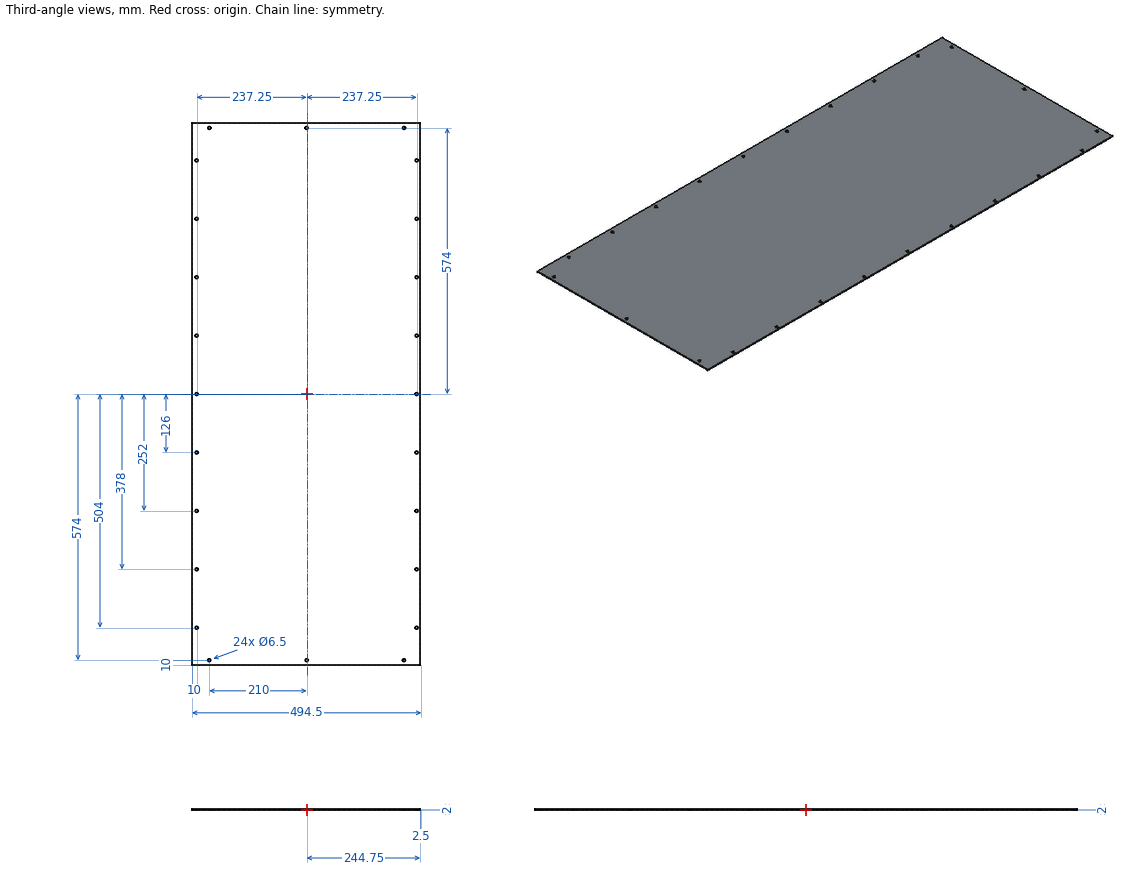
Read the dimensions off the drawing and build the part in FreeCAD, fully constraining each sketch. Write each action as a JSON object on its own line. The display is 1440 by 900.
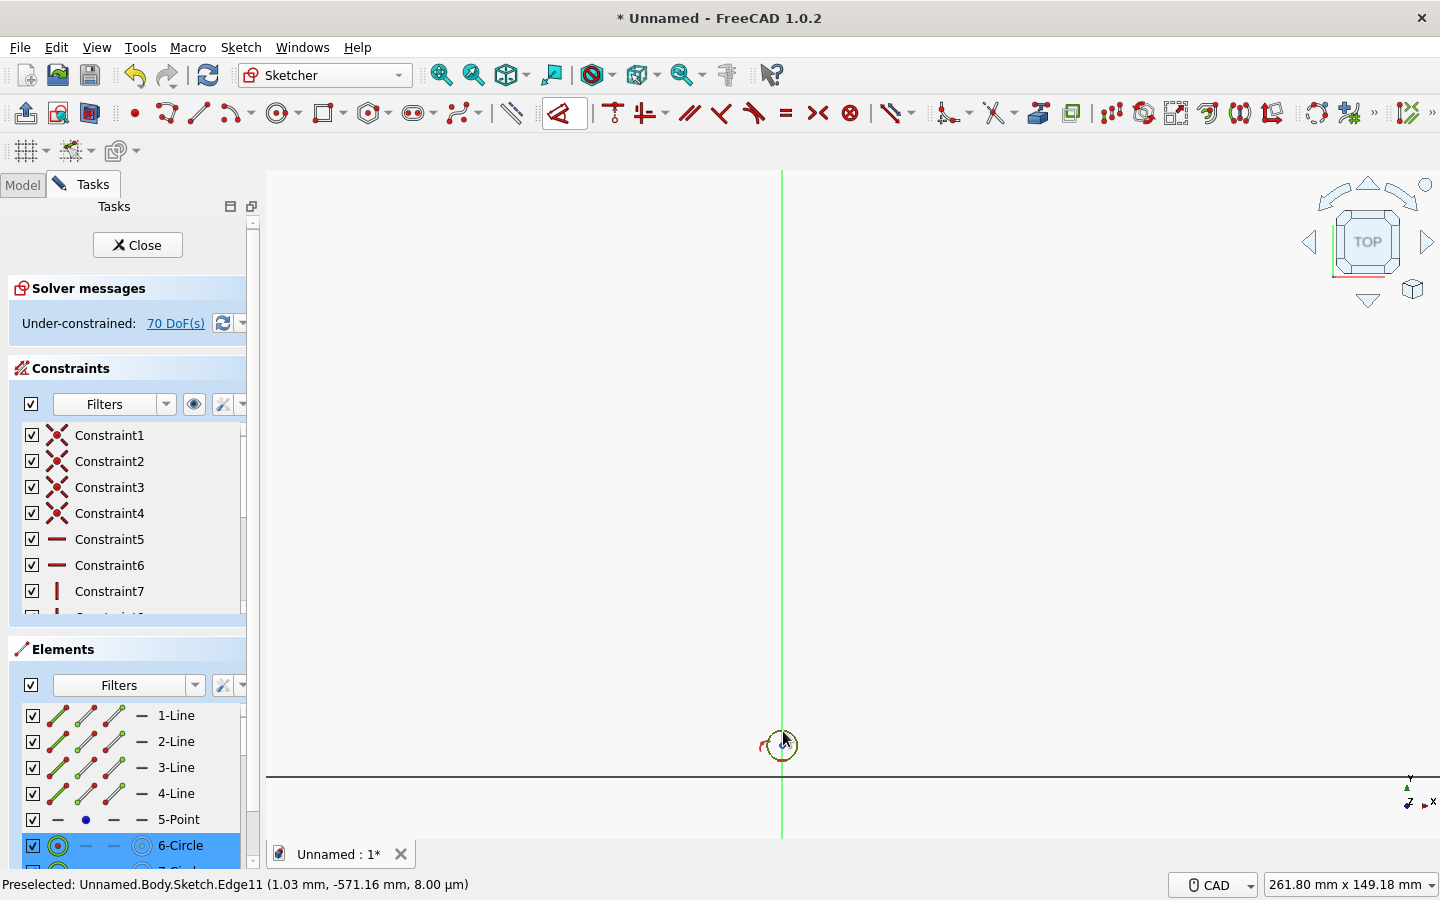
{"action": "scroll", "coordinate": [785, 737], "scroll_direction": "down", "scroll_amount": 12}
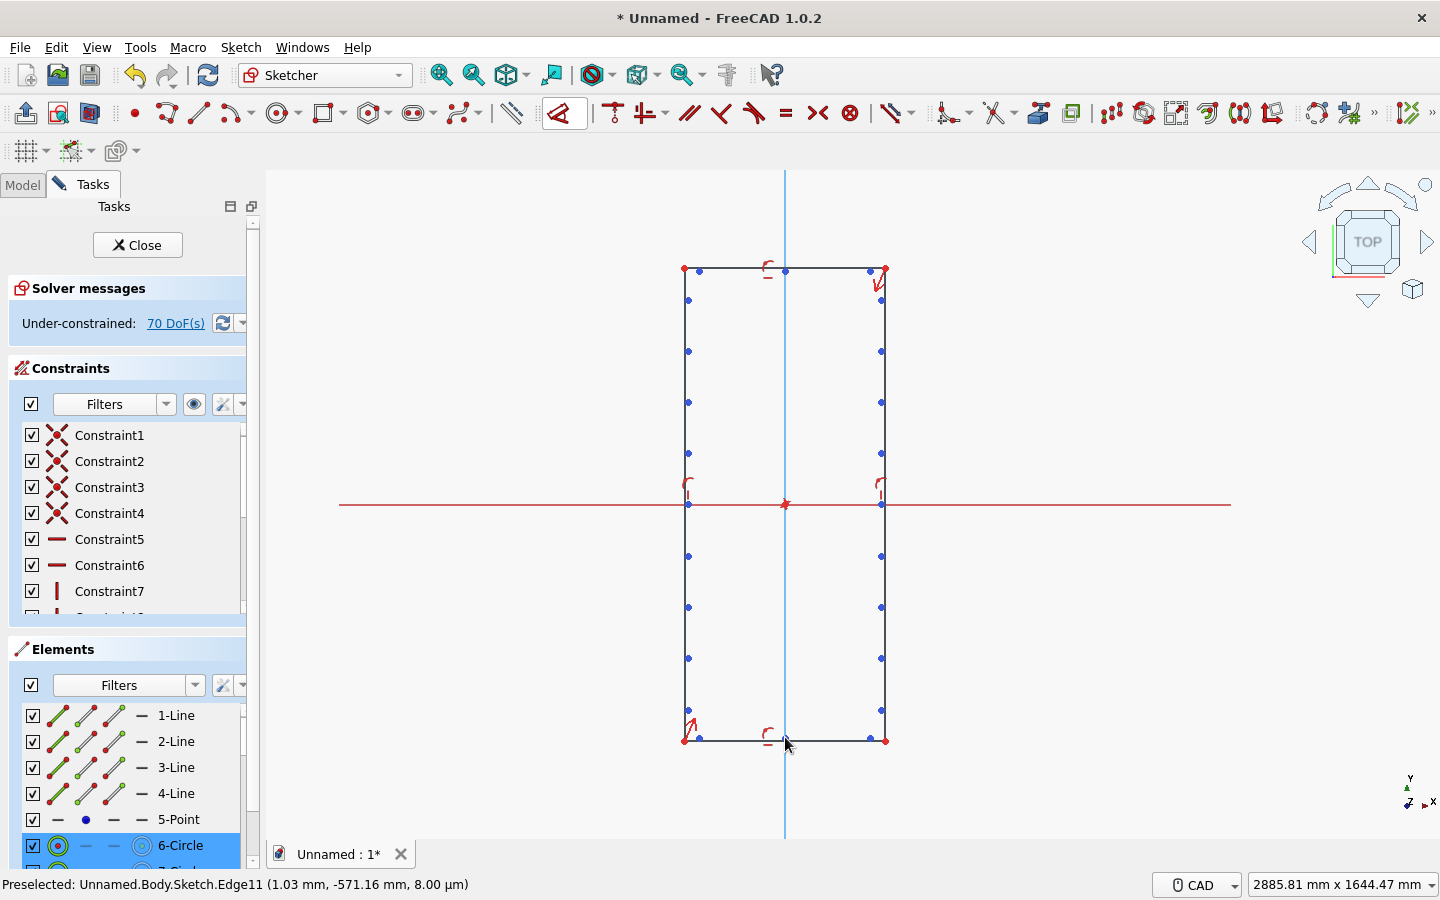
{"action": "scroll", "coordinate": [872, 738], "scroll_direction": "up", "scroll_amount": 12}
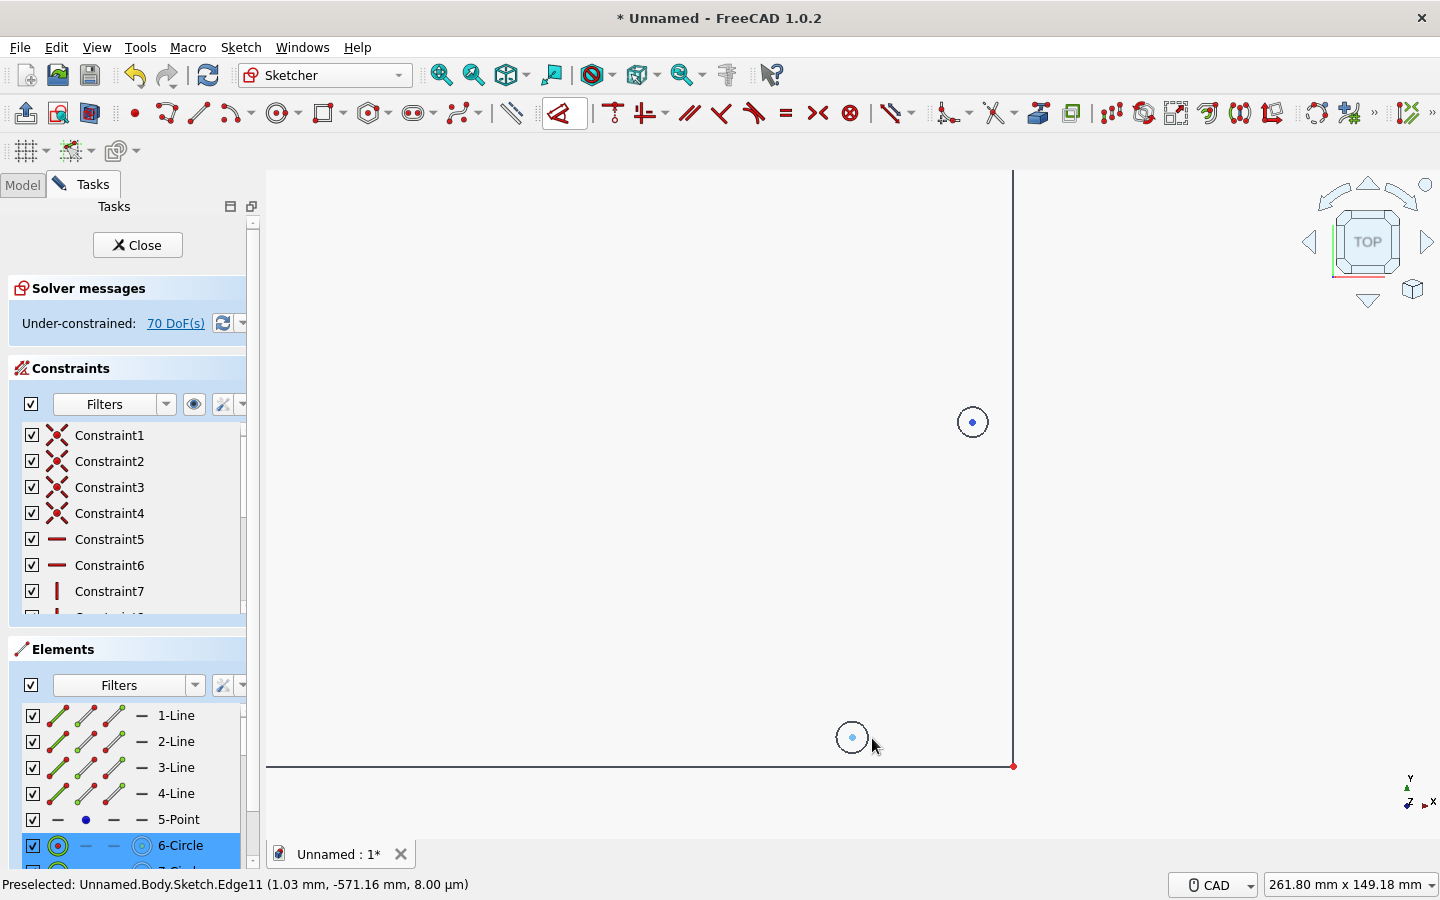
{"action": "left_click", "coordinate": [863, 726]}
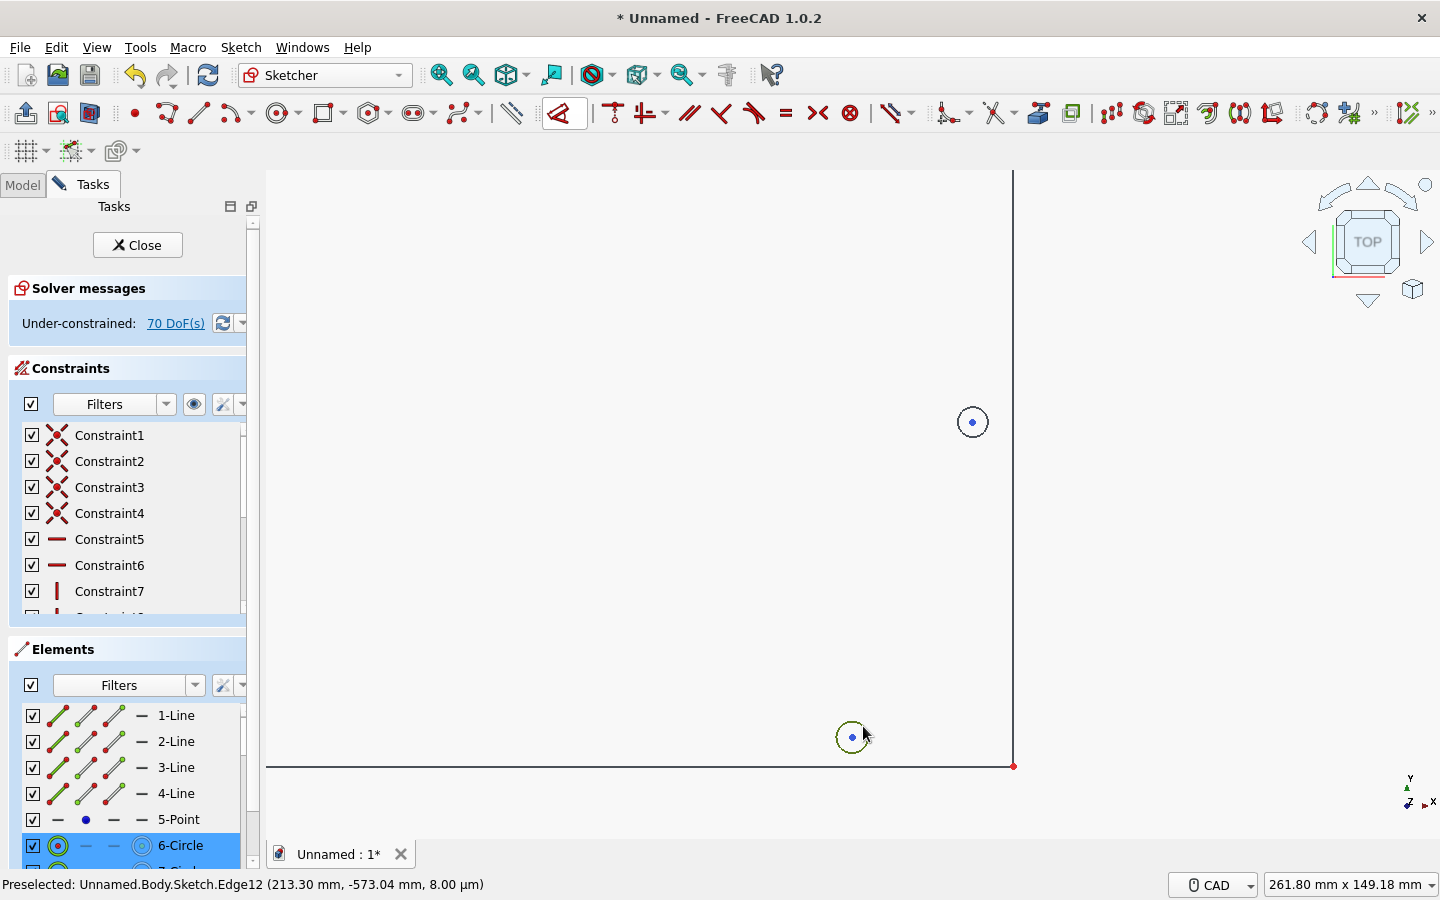
{"action": "left_click", "coordinate": [983, 411]}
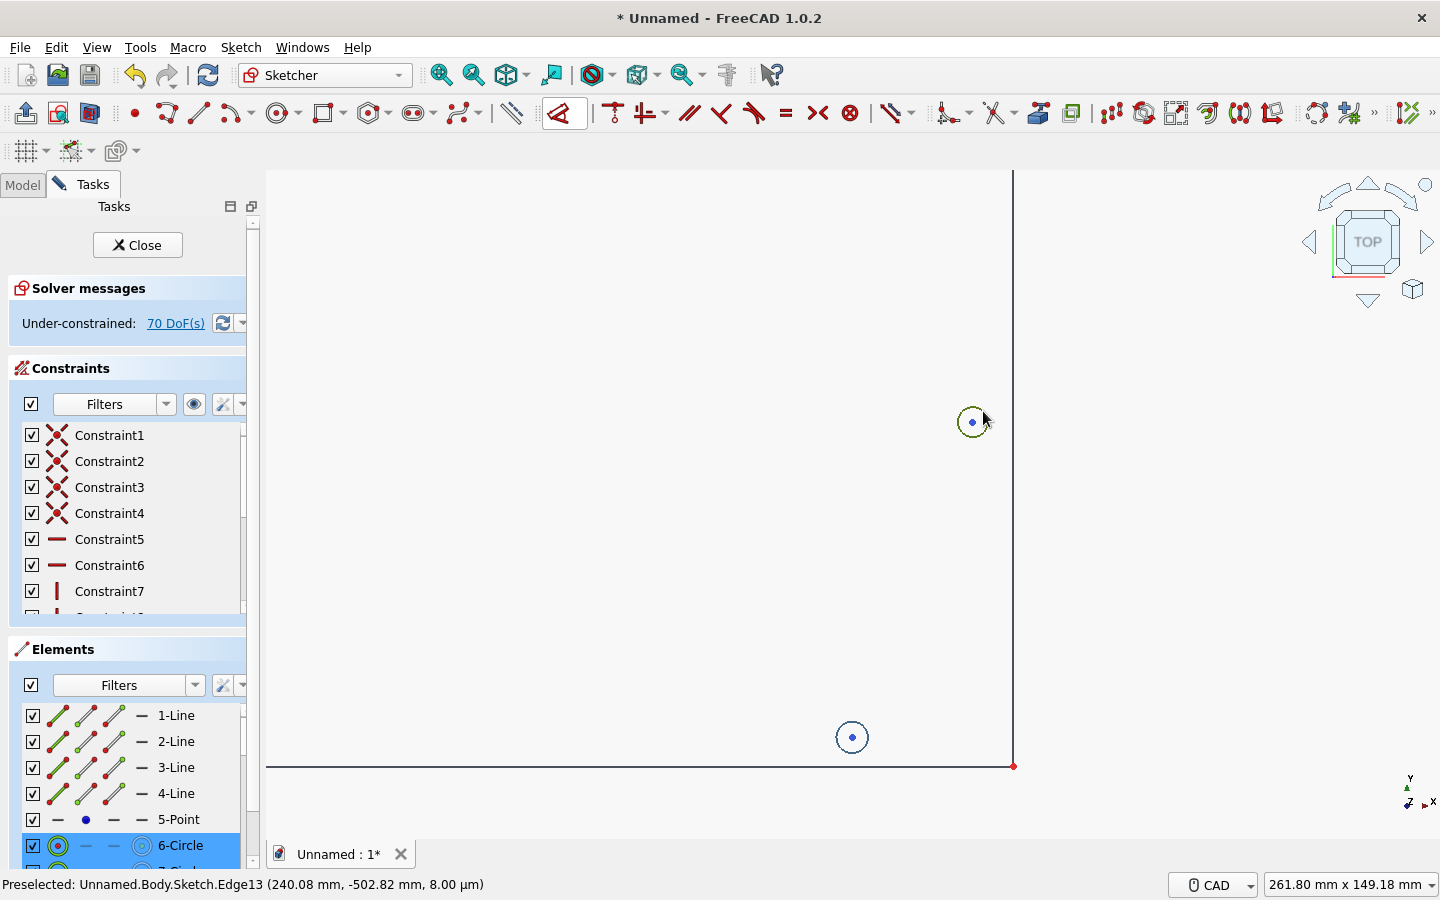
{"action": "scroll", "coordinate": [872, 738], "scroll_direction": "down", "scroll_amount": 12}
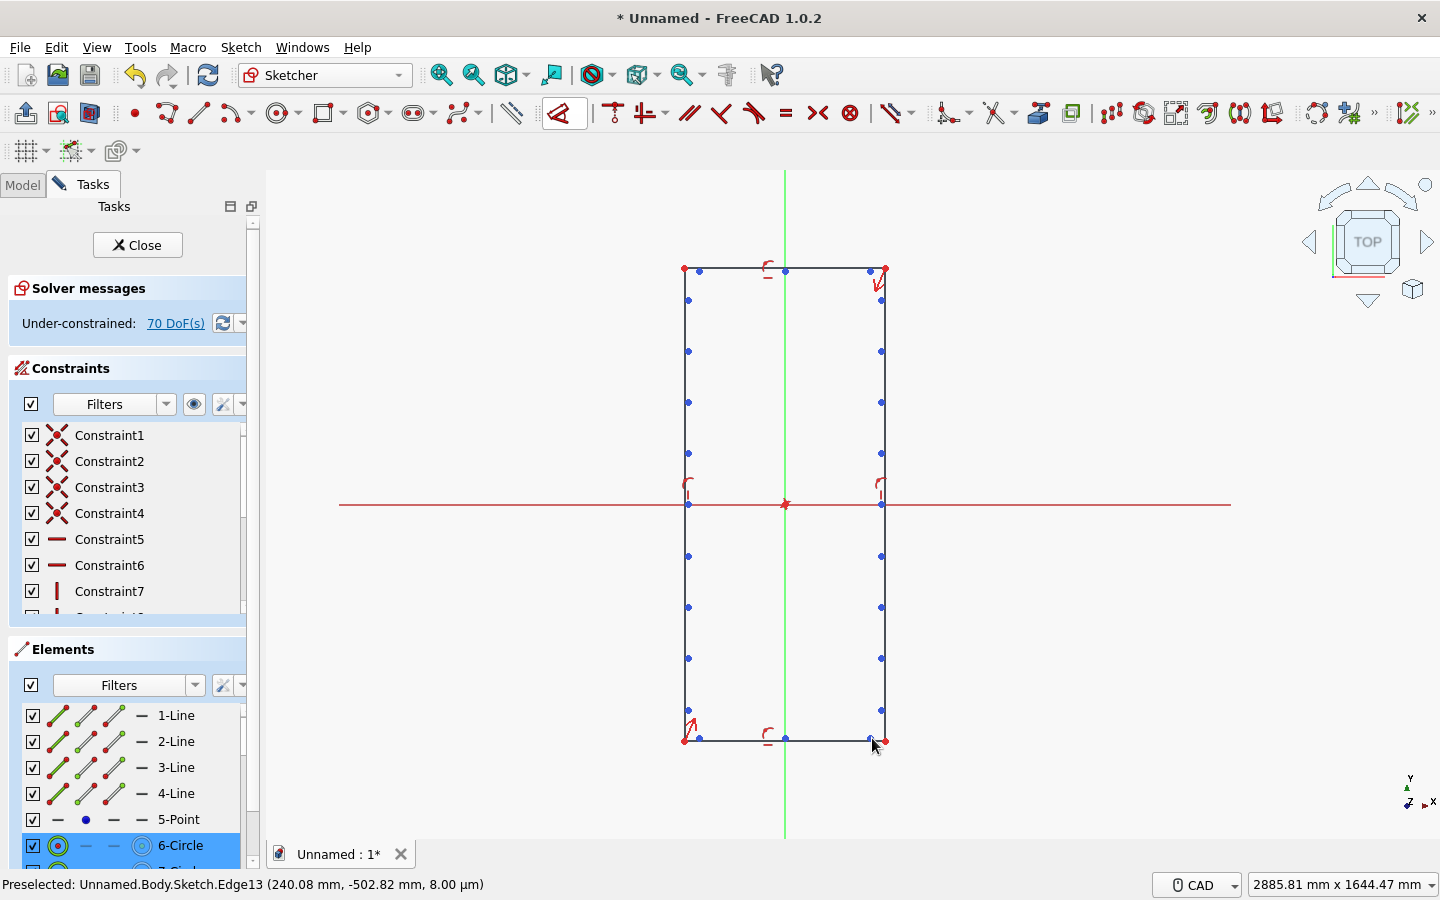
{"action": "scroll", "coordinate": [883, 658], "scroll_direction": "up", "scroll_amount": 12}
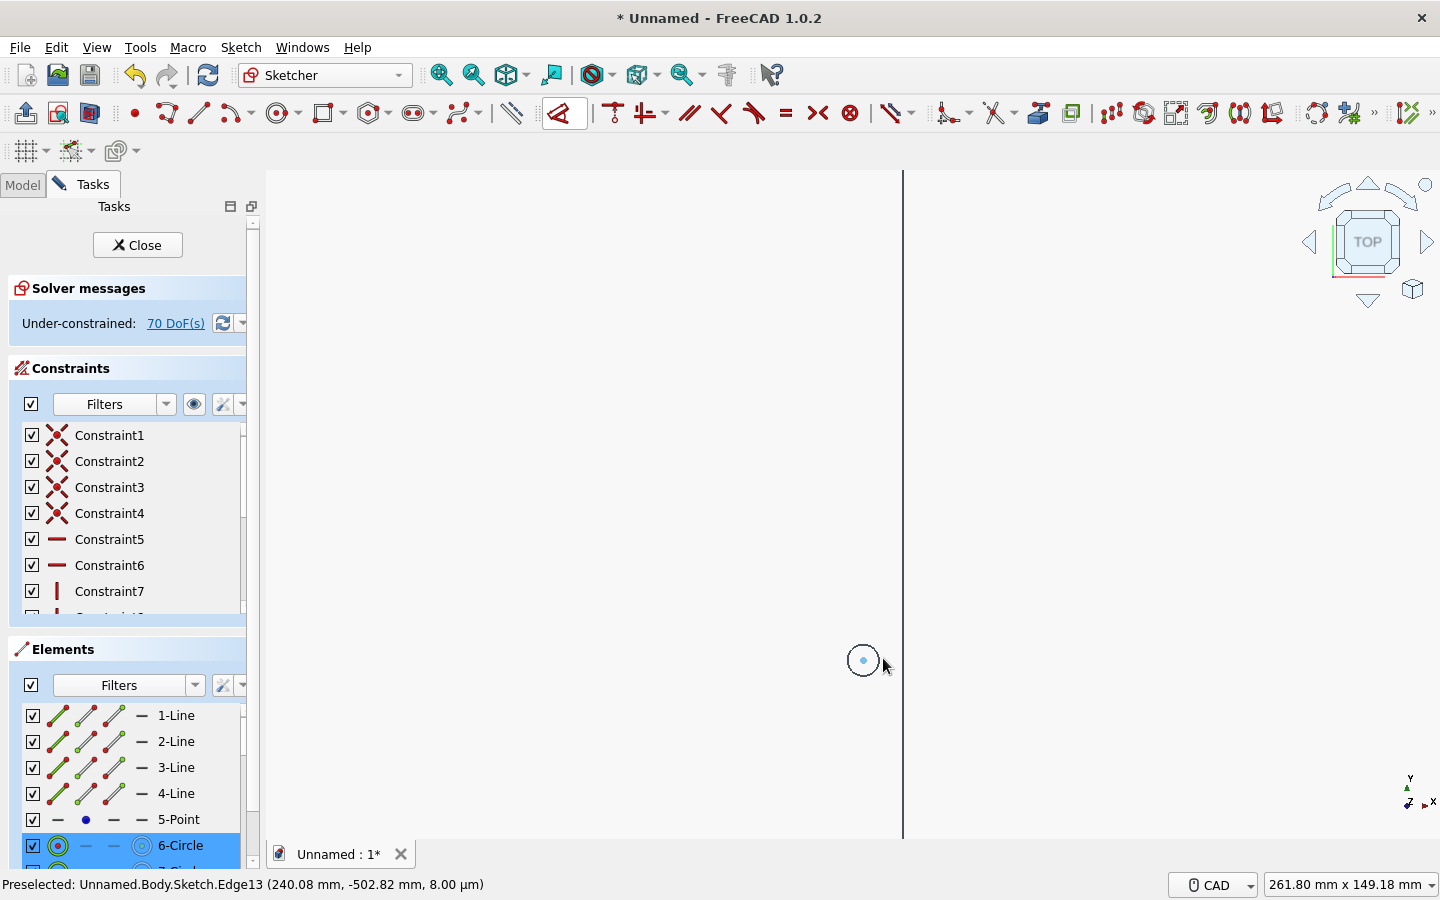
{"action": "left_click", "coordinate": [874, 649]}